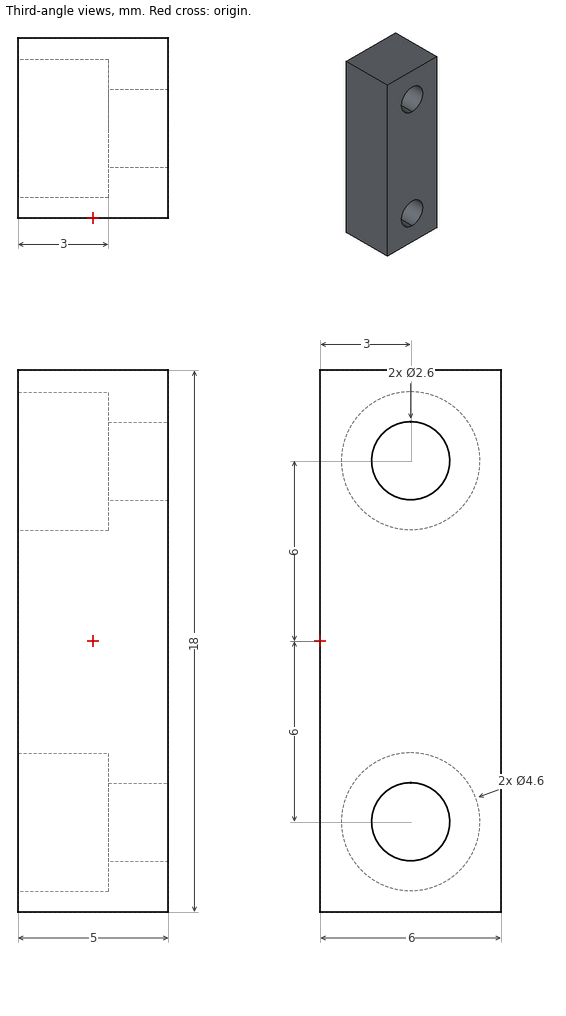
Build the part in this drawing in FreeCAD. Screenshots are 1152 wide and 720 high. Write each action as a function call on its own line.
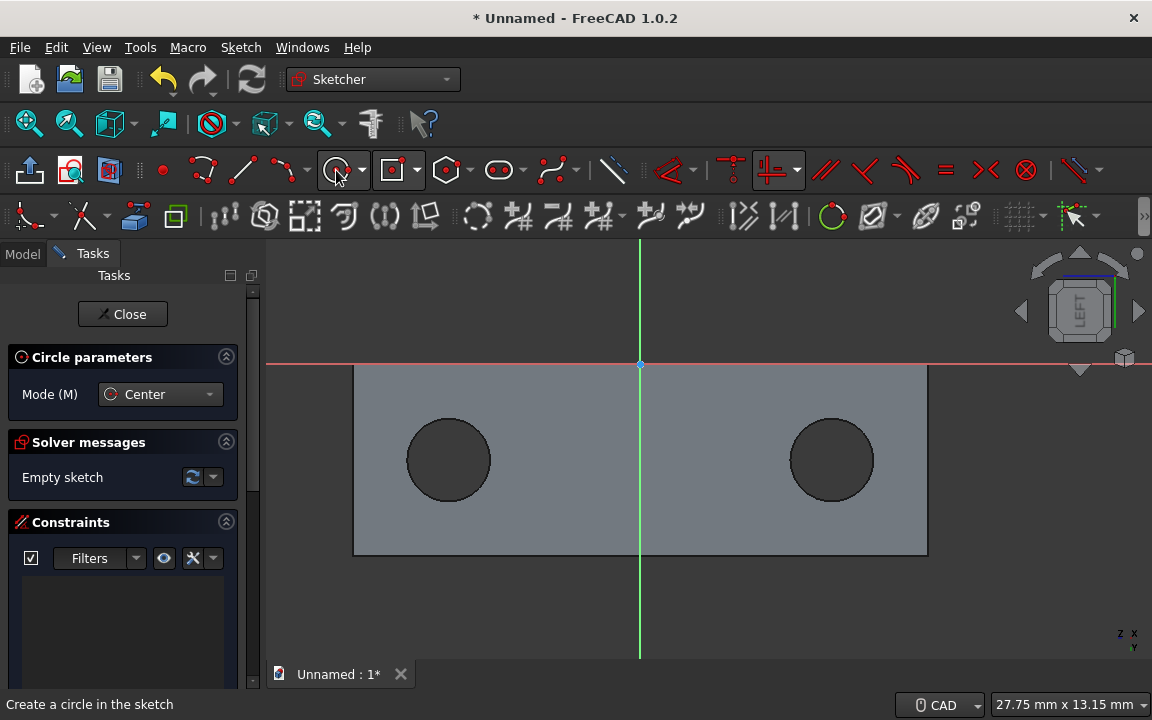
click(832, 460)
click(884, 408)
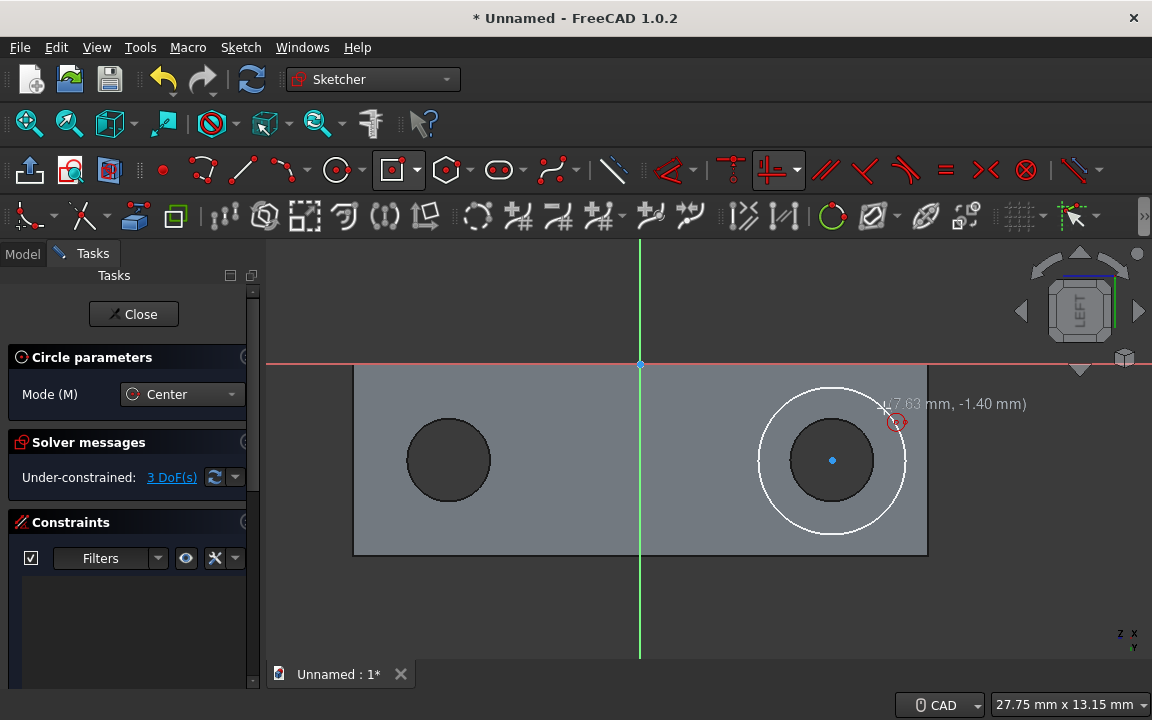
click(449, 460)
click(501, 408)
key(Escape)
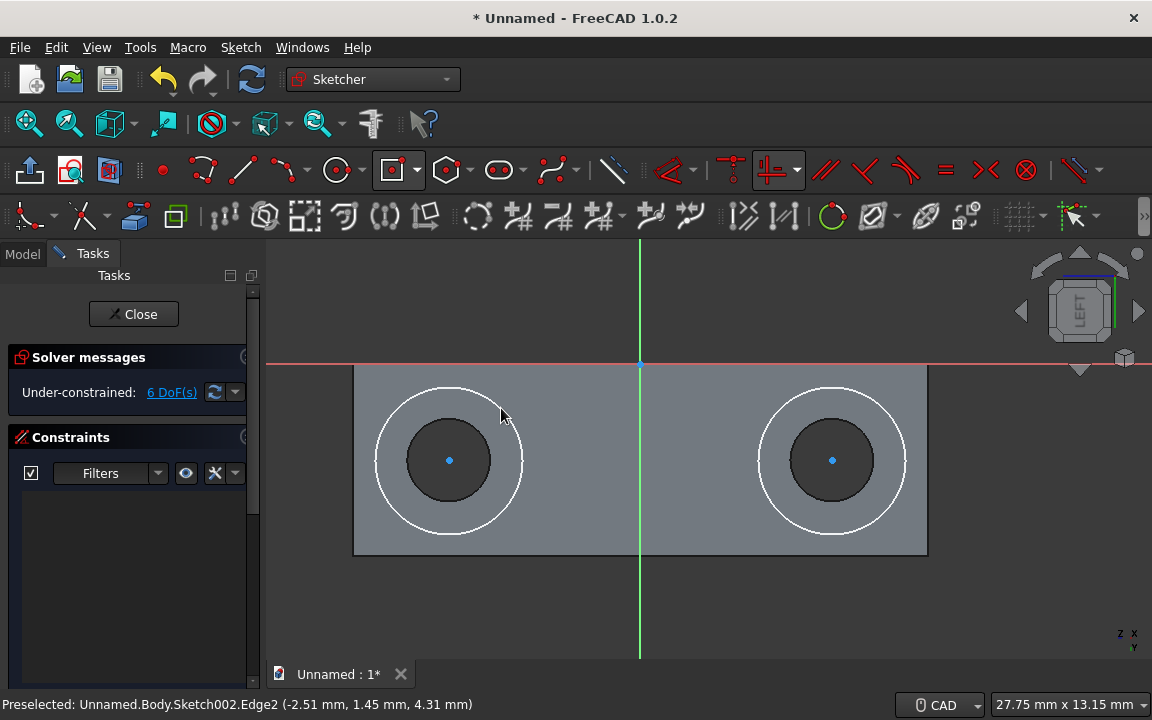
click(884, 409)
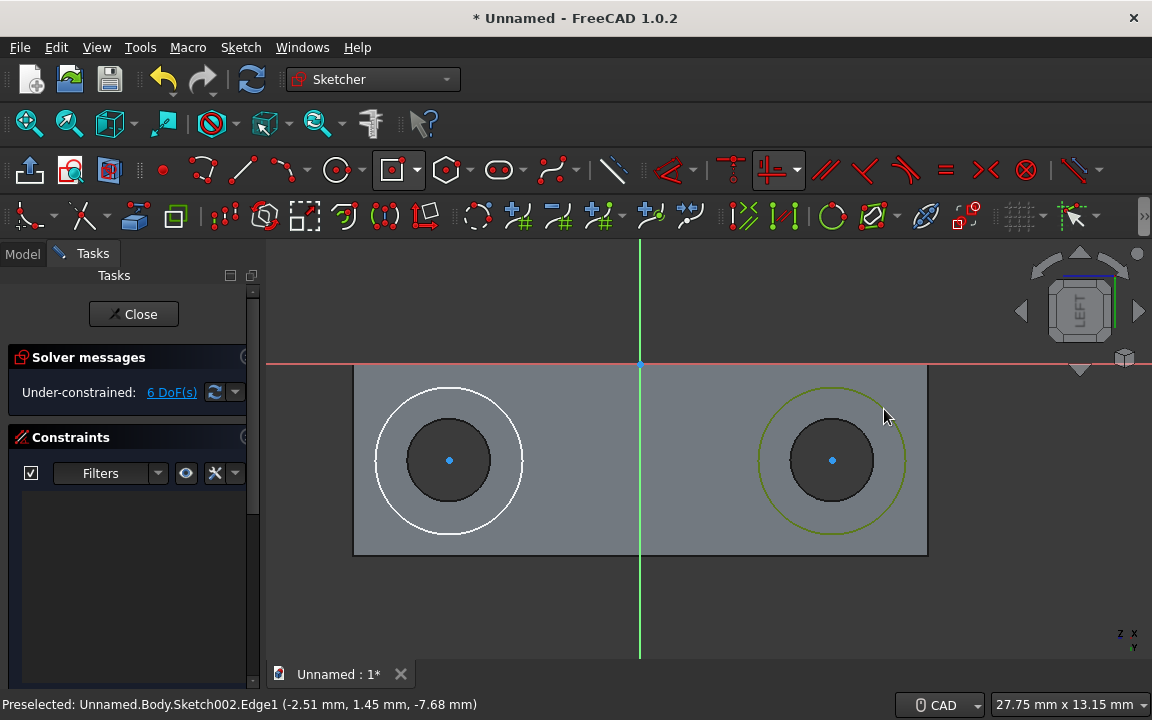
click(501, 409)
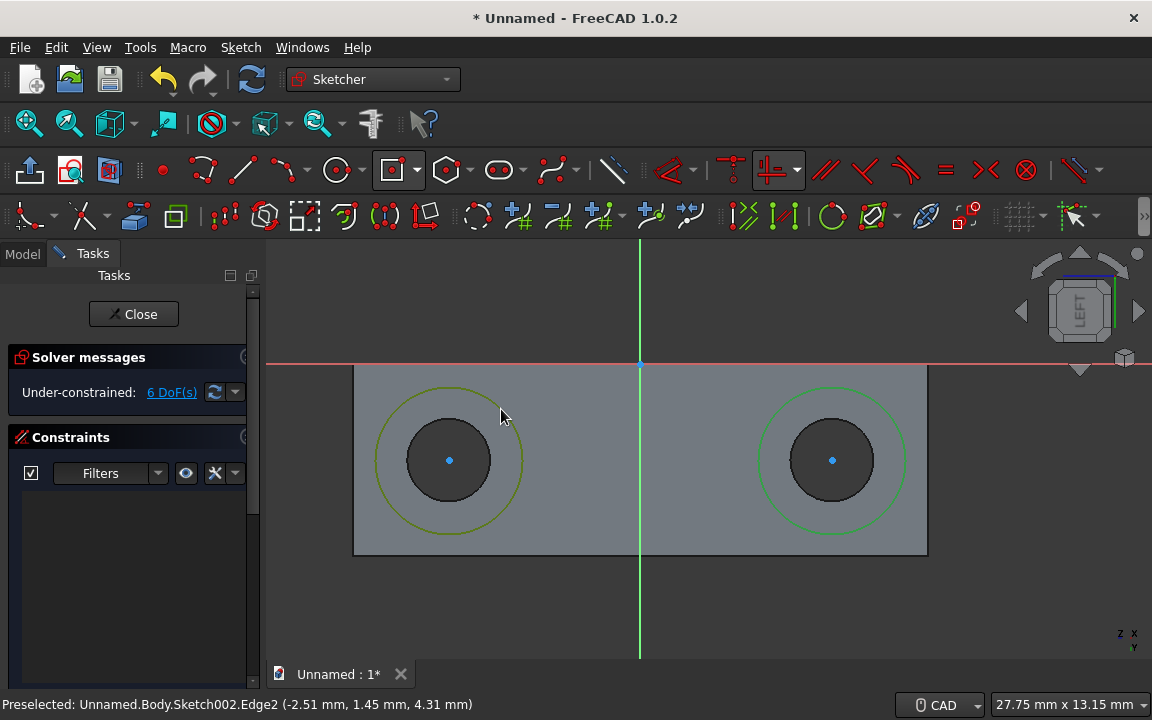
click(946, 170)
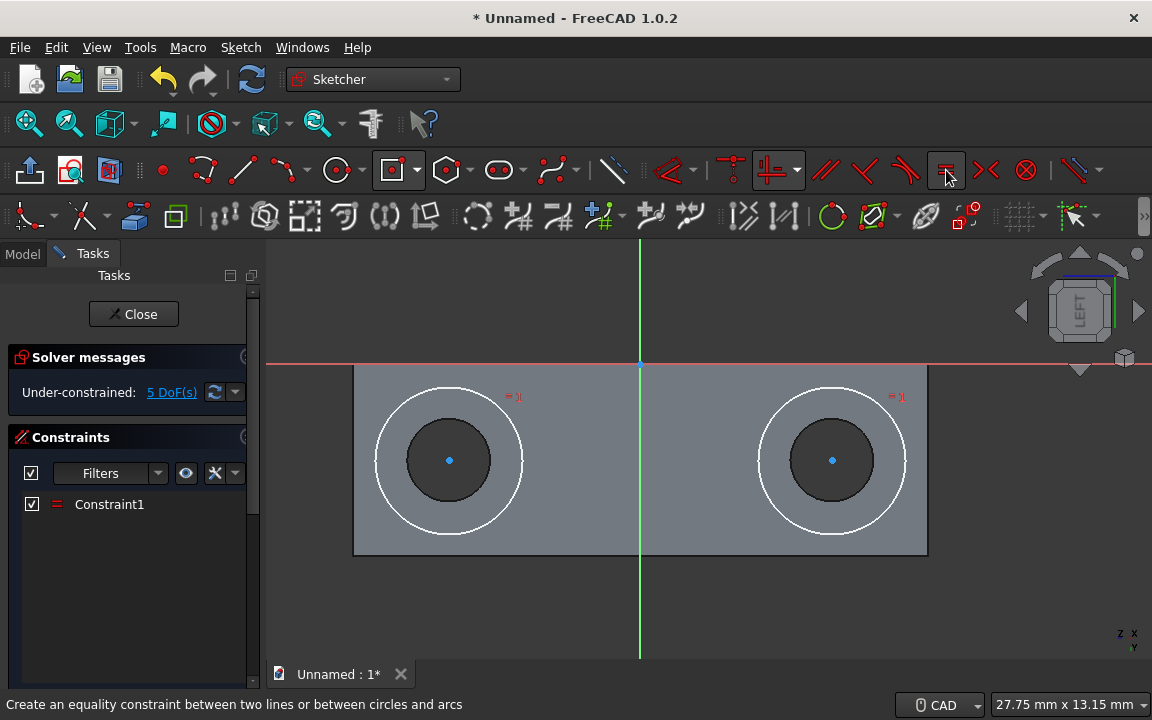
click(832, 461)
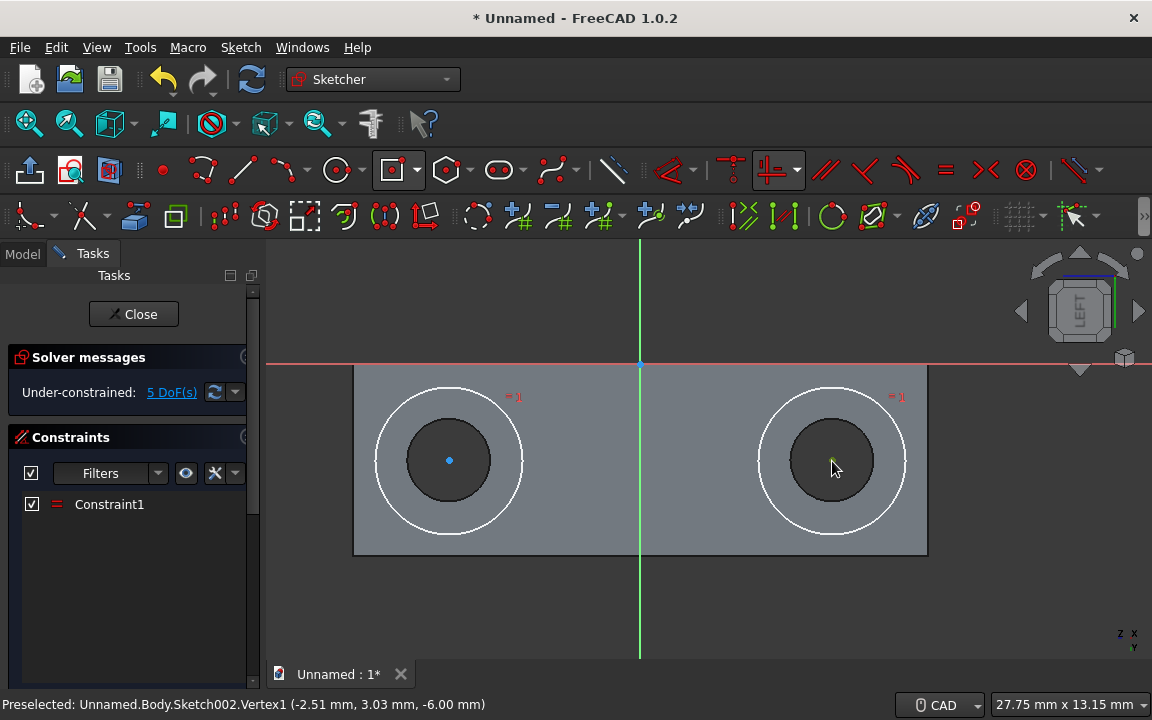
click(449, 461)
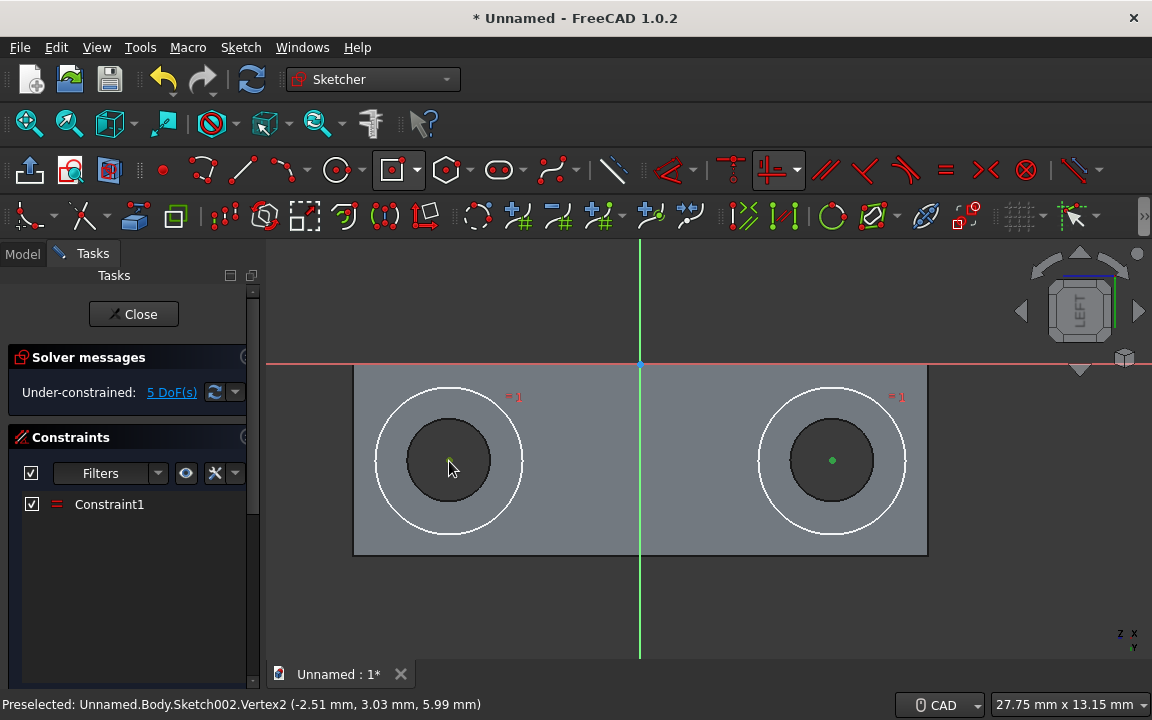
key(h)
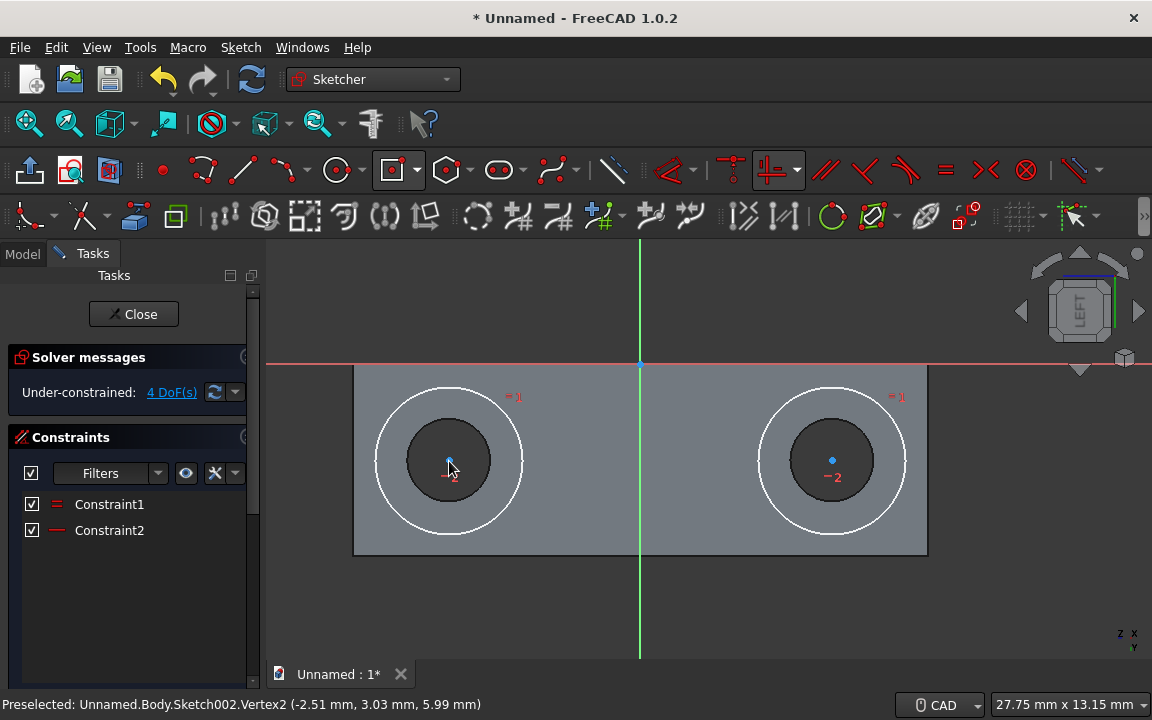
click(668, 170)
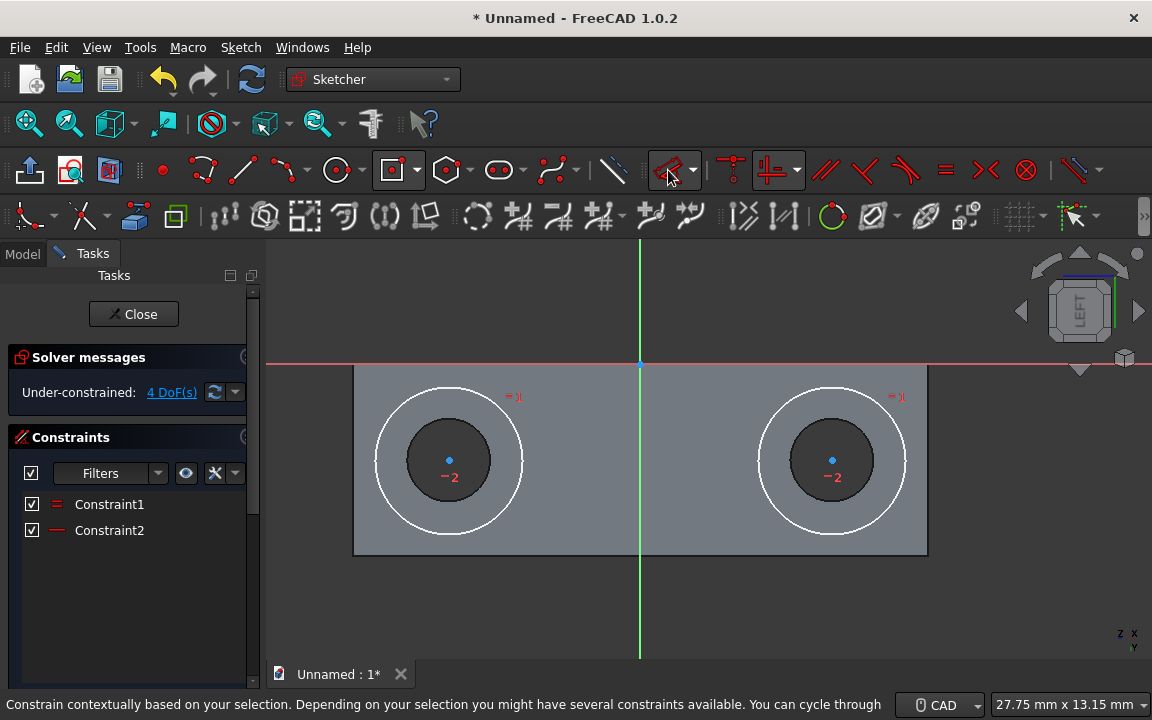
click(884, 409)
click(907, 386)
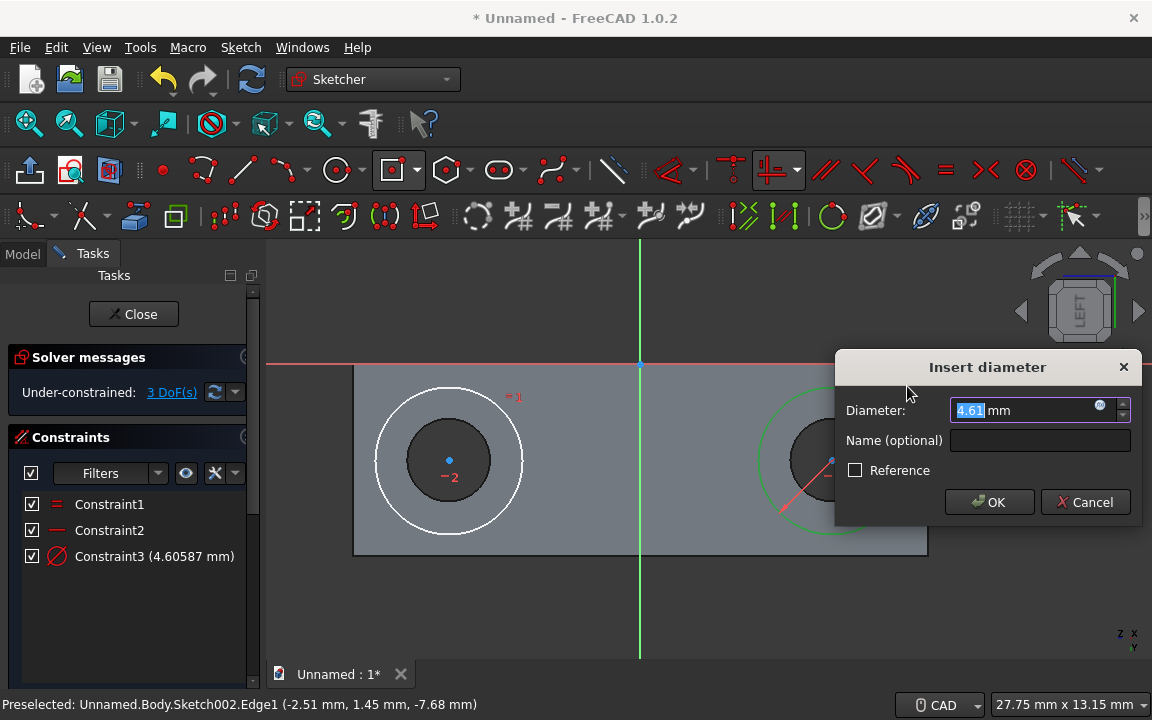
text(4.6)
key(Return)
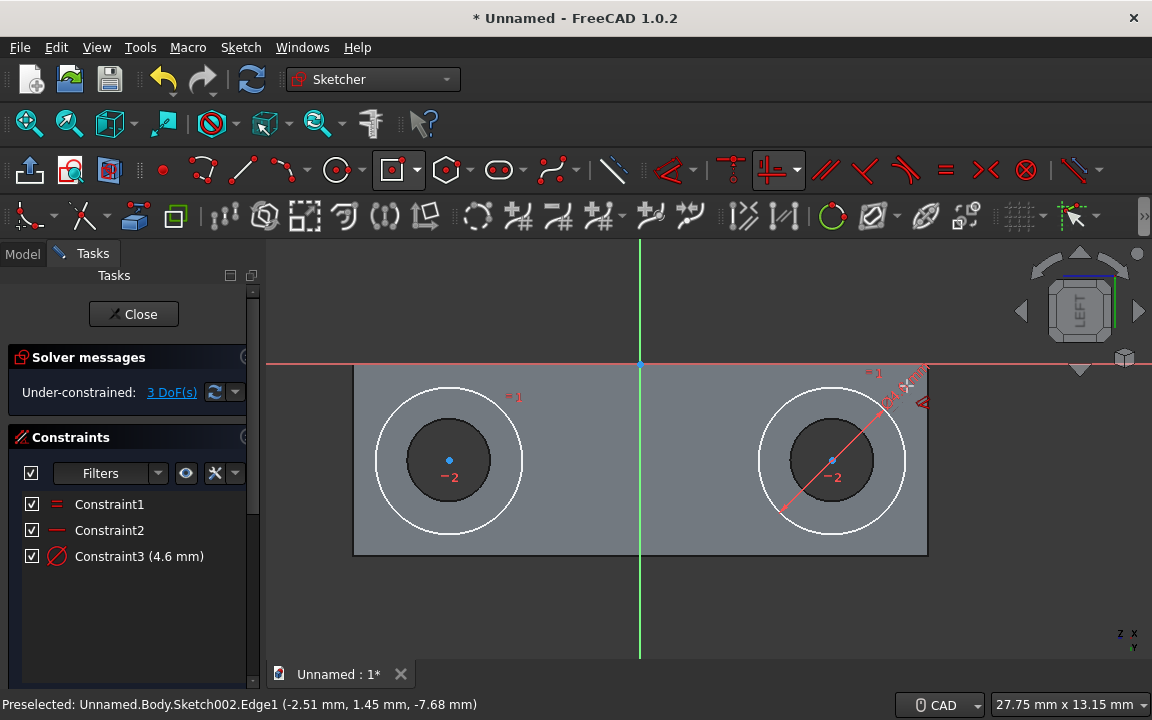
click(832, 461)
click(736, 330)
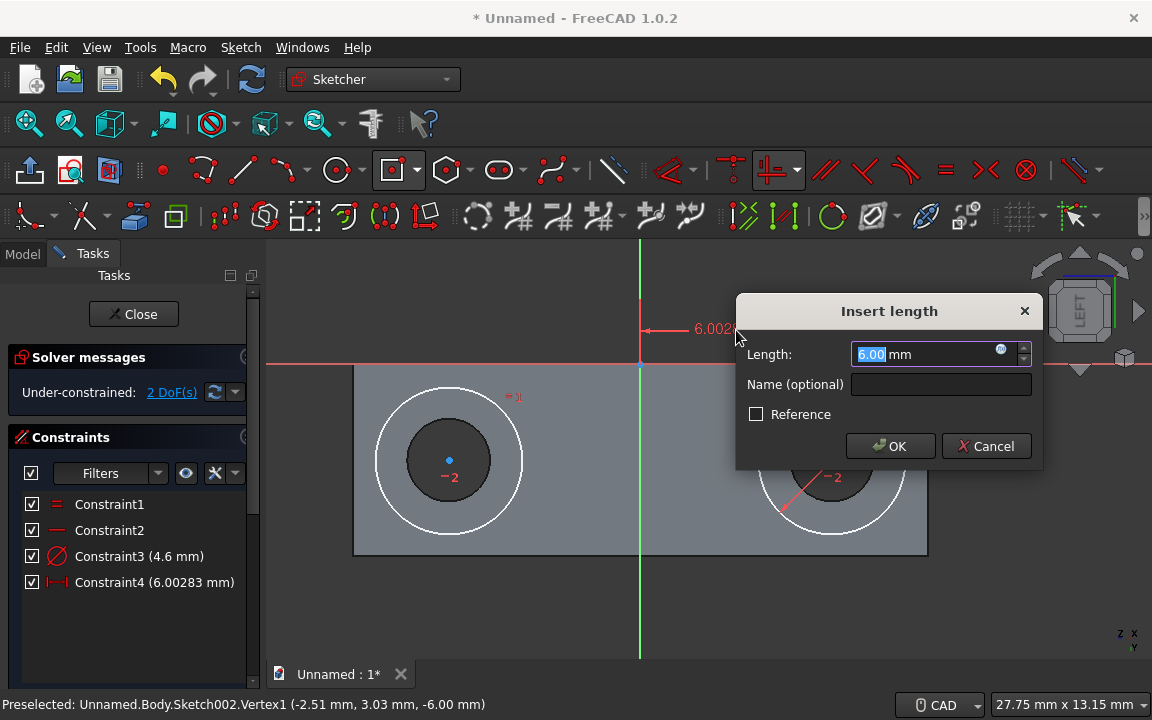
text(6)
key(Return)